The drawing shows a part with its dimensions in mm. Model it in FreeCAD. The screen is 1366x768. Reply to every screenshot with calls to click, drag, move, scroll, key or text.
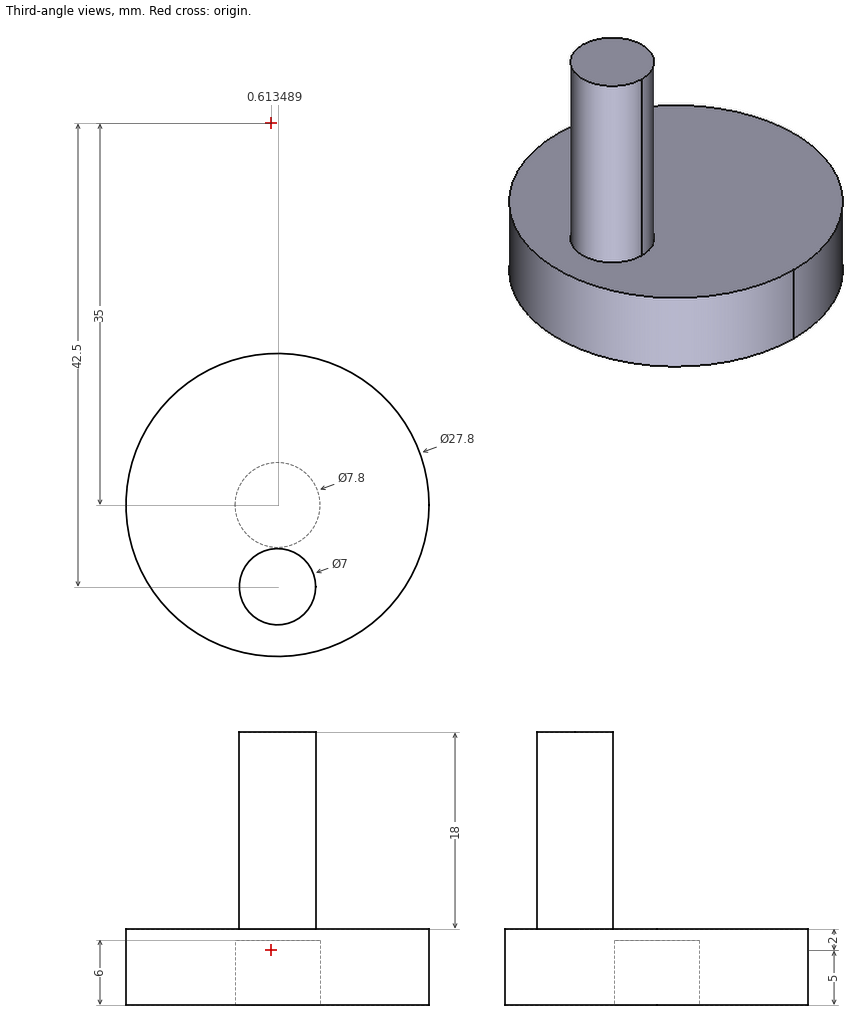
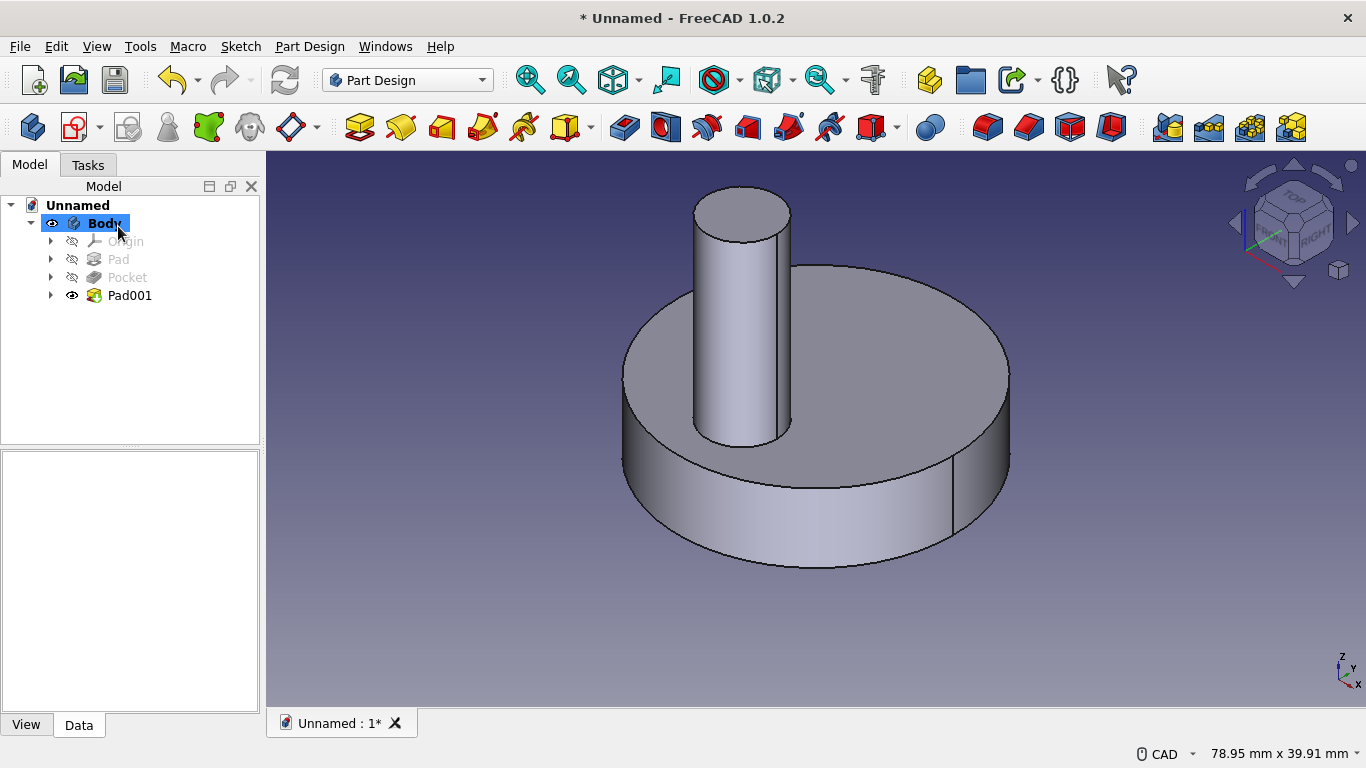
click(531, 80)